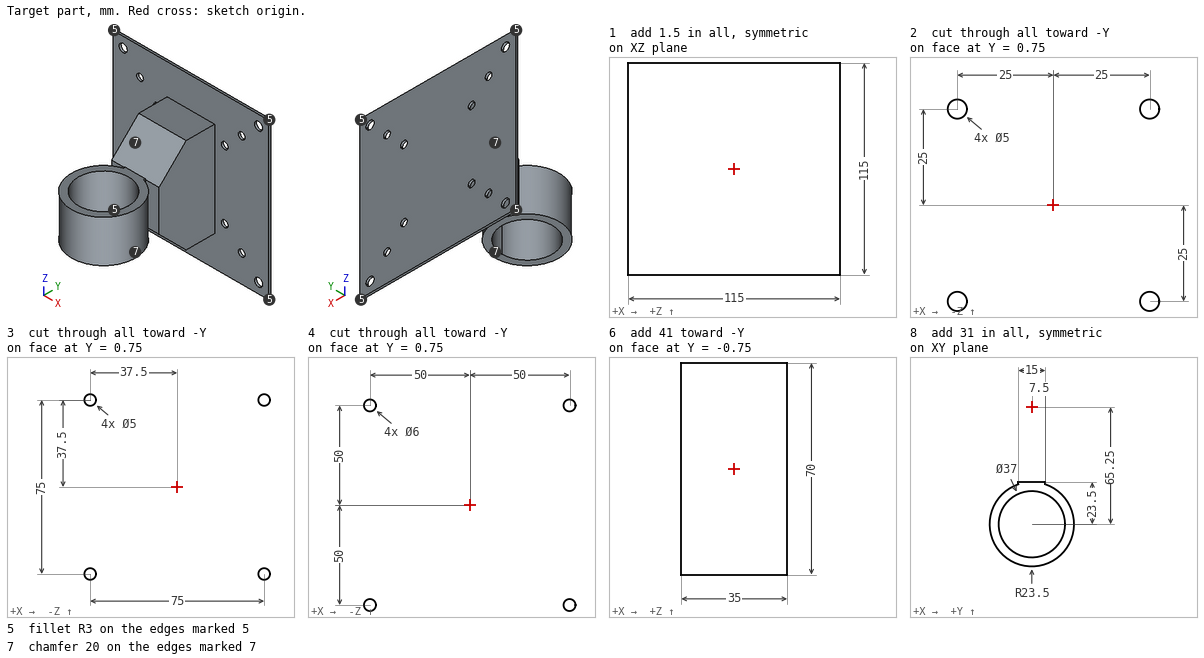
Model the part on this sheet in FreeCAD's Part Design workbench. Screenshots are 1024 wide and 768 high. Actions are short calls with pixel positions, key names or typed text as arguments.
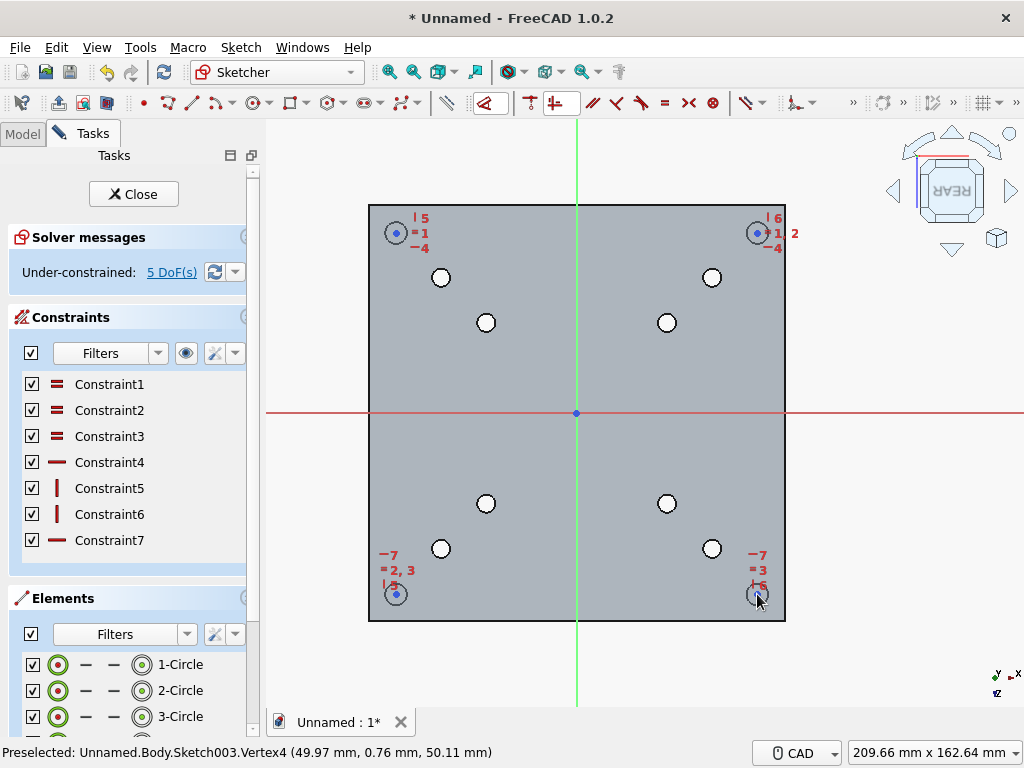
key(d)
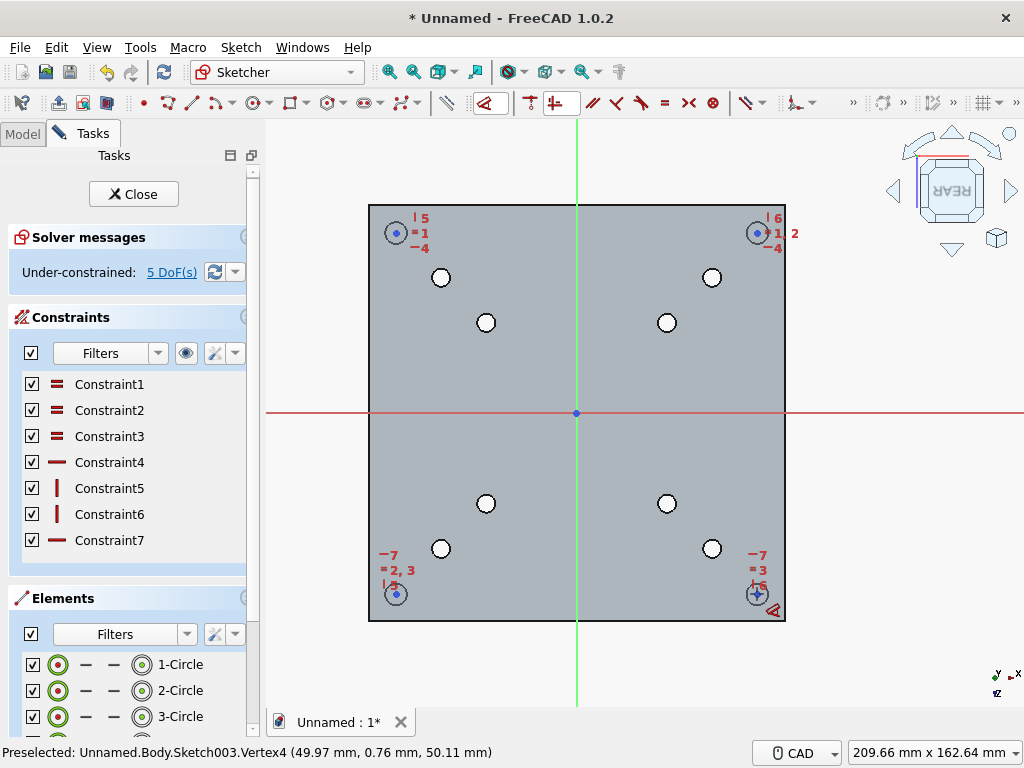
scroll(404, 225, up, 4)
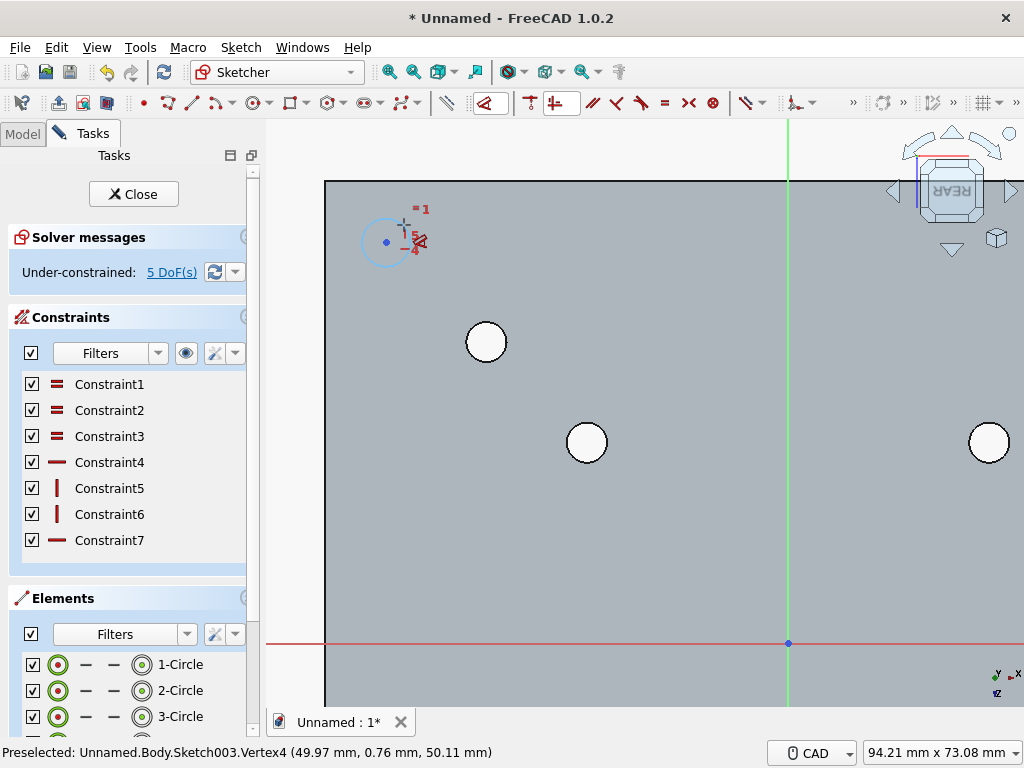
click(403, 226)
click(426, 203)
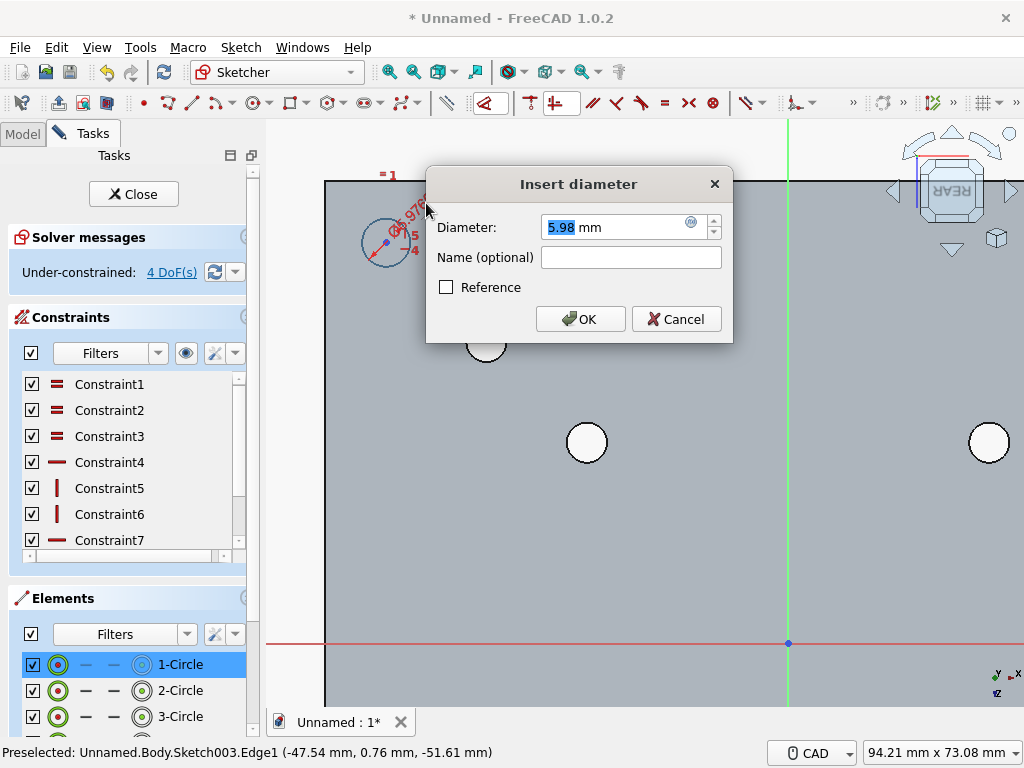
text(6)
key(Return)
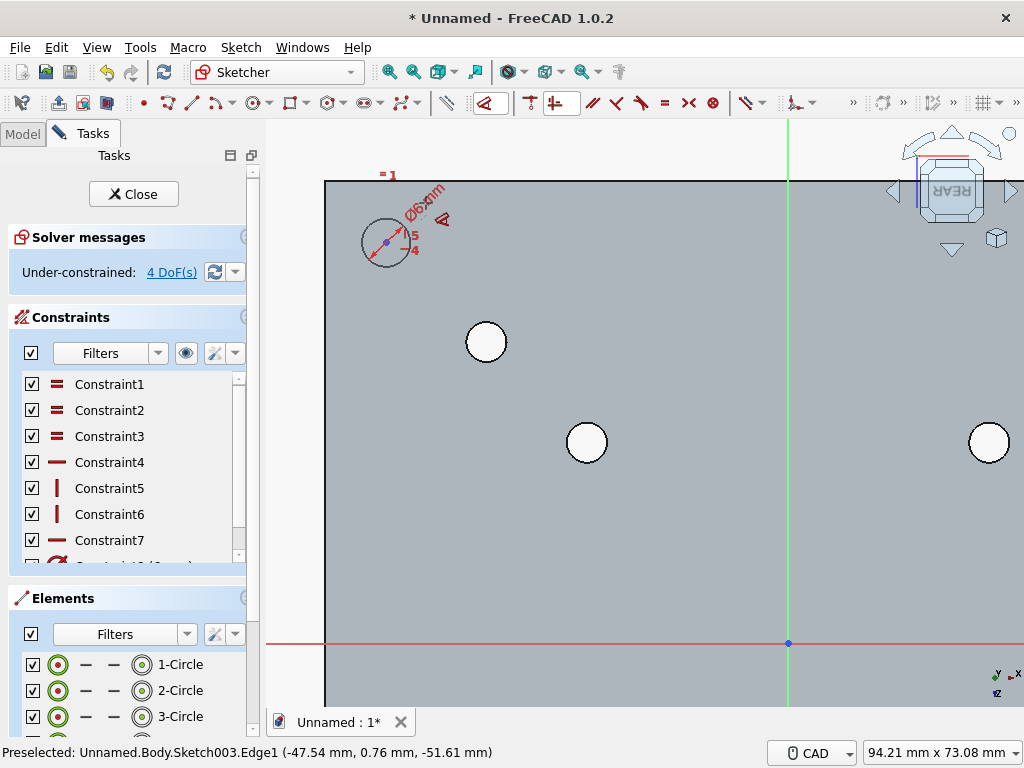
click(386, 243)
click(587, 209)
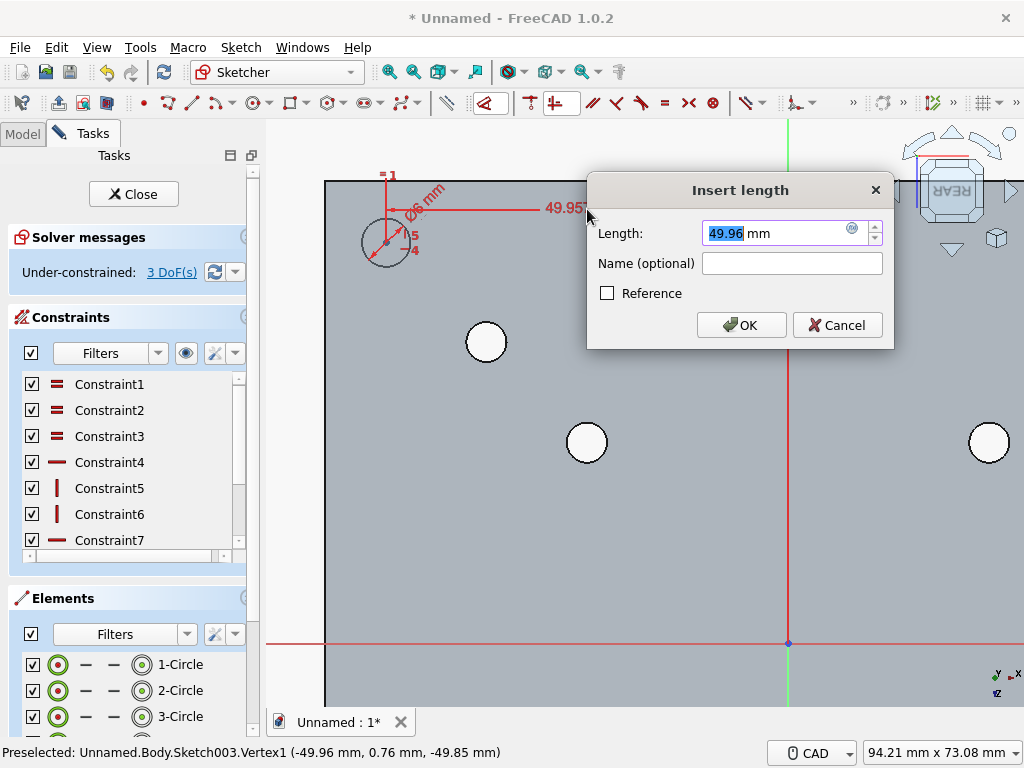
text(50)
key(Return)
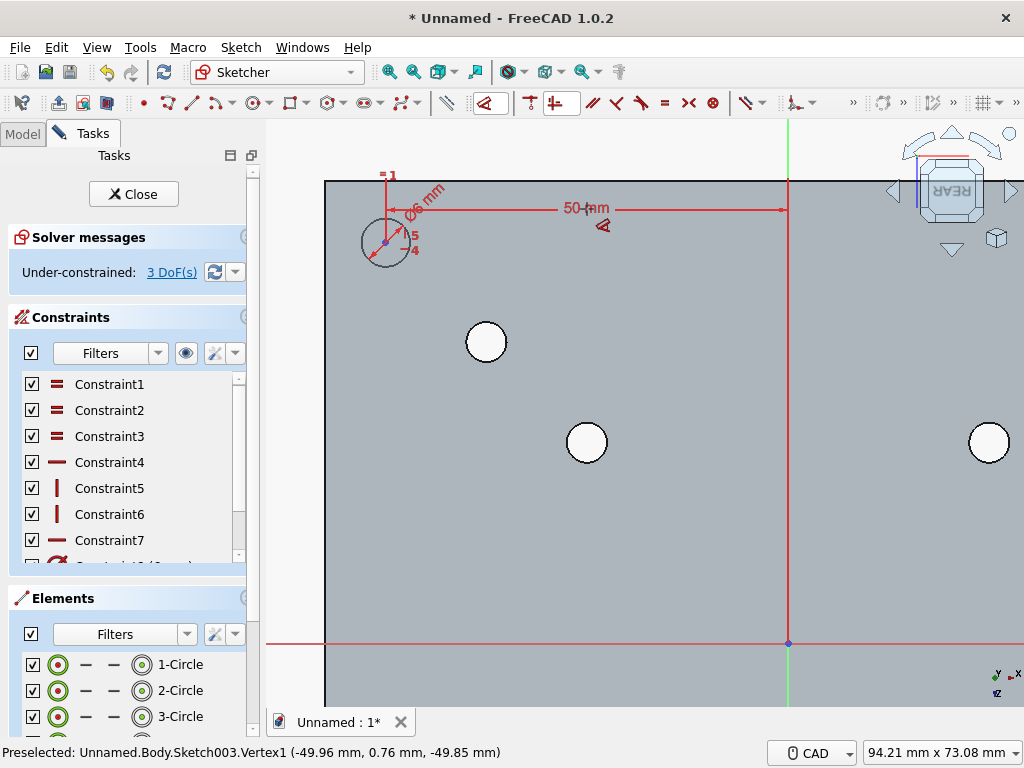
click(386, 243)
click(352, 443)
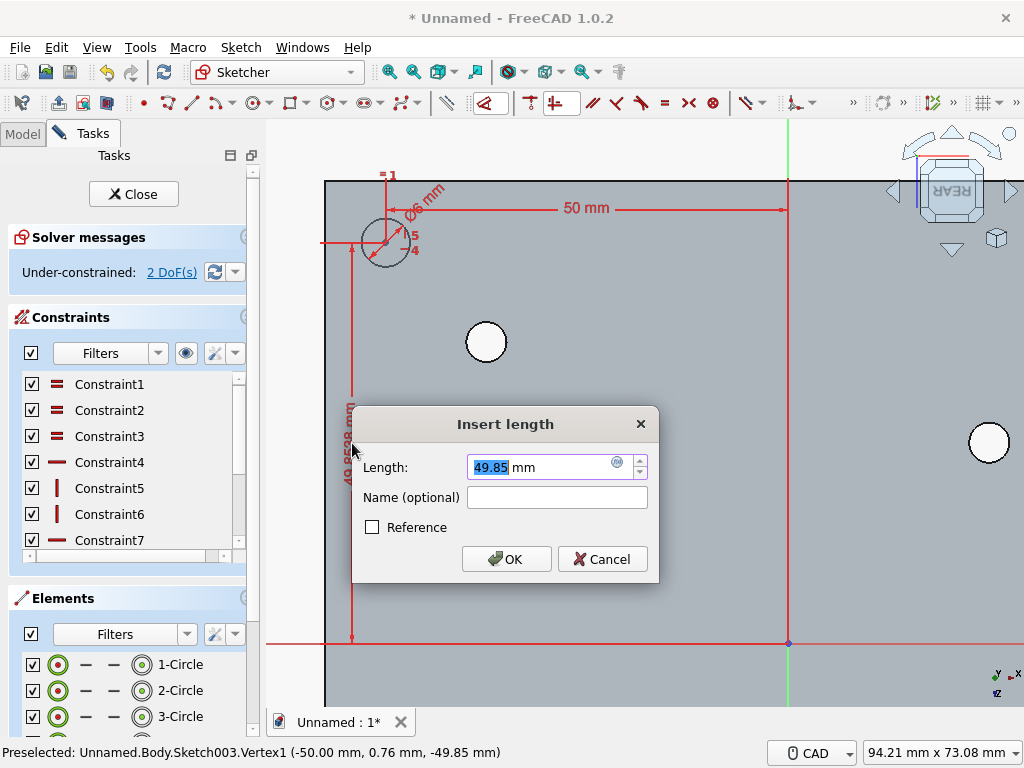
text(50)
key(Return)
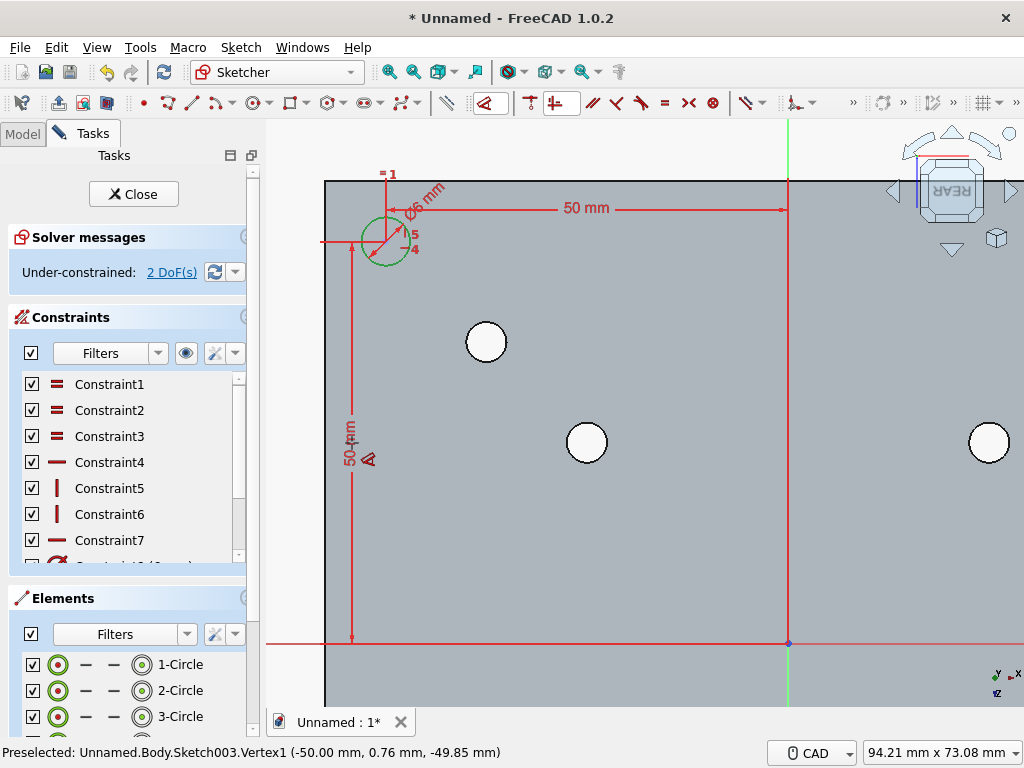
scroll(404, 225, down, 4)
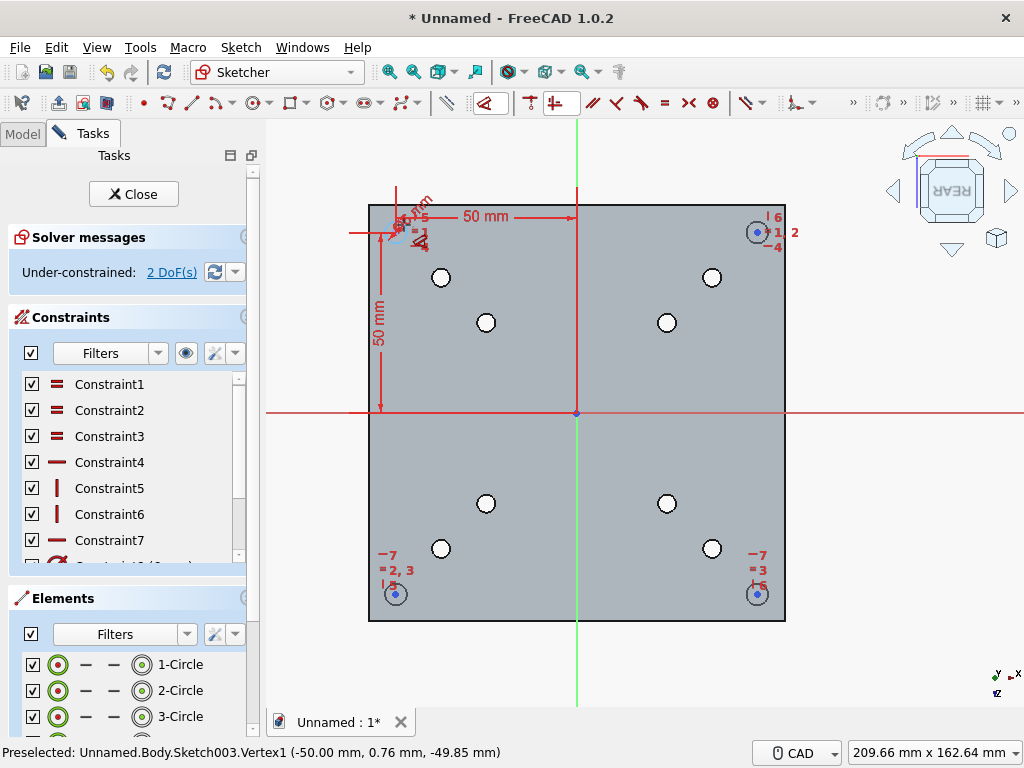
click(757, 233)
click(667, 199)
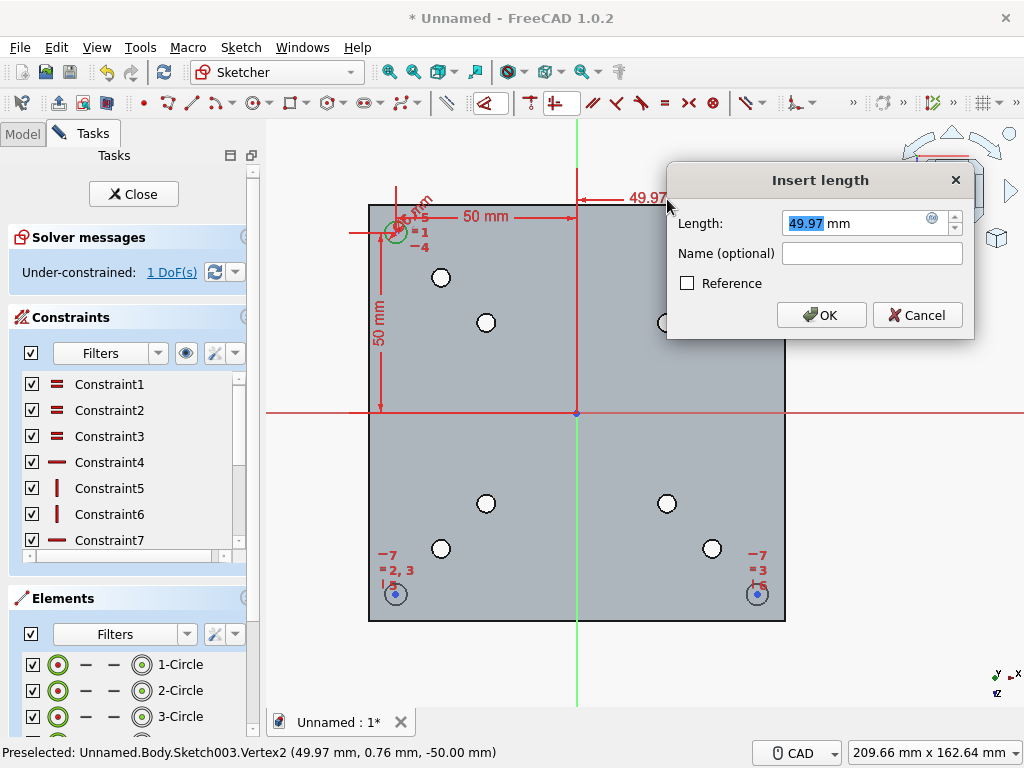
text(50)
key(Return)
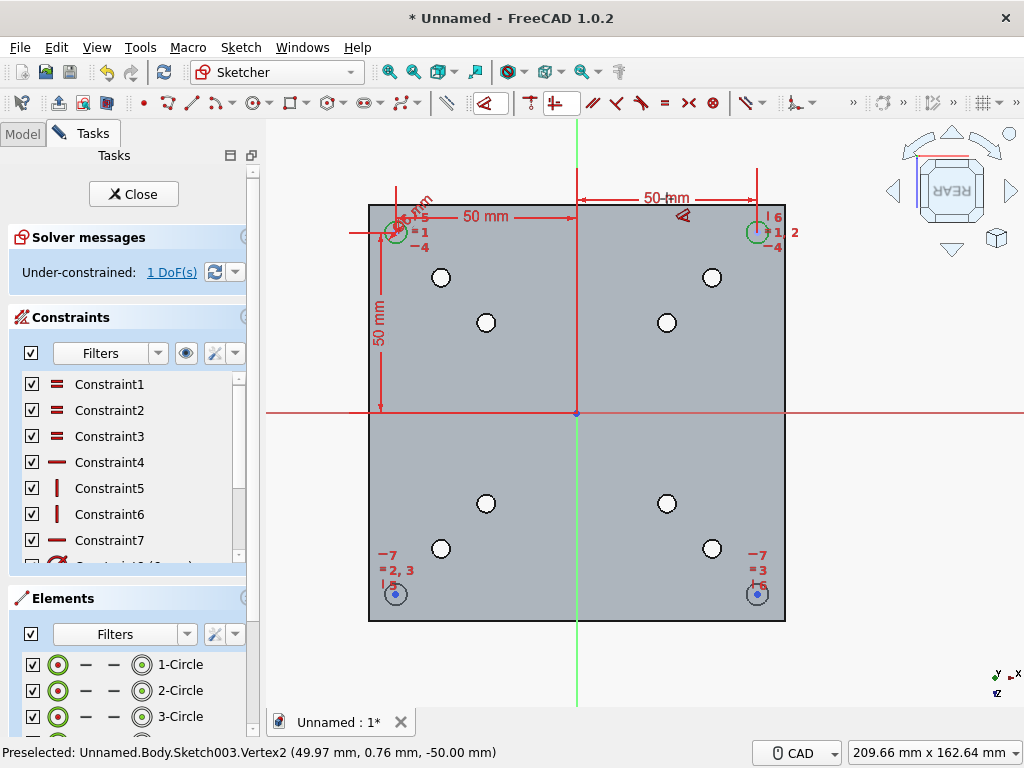
click(396, 594)
click(362, 504)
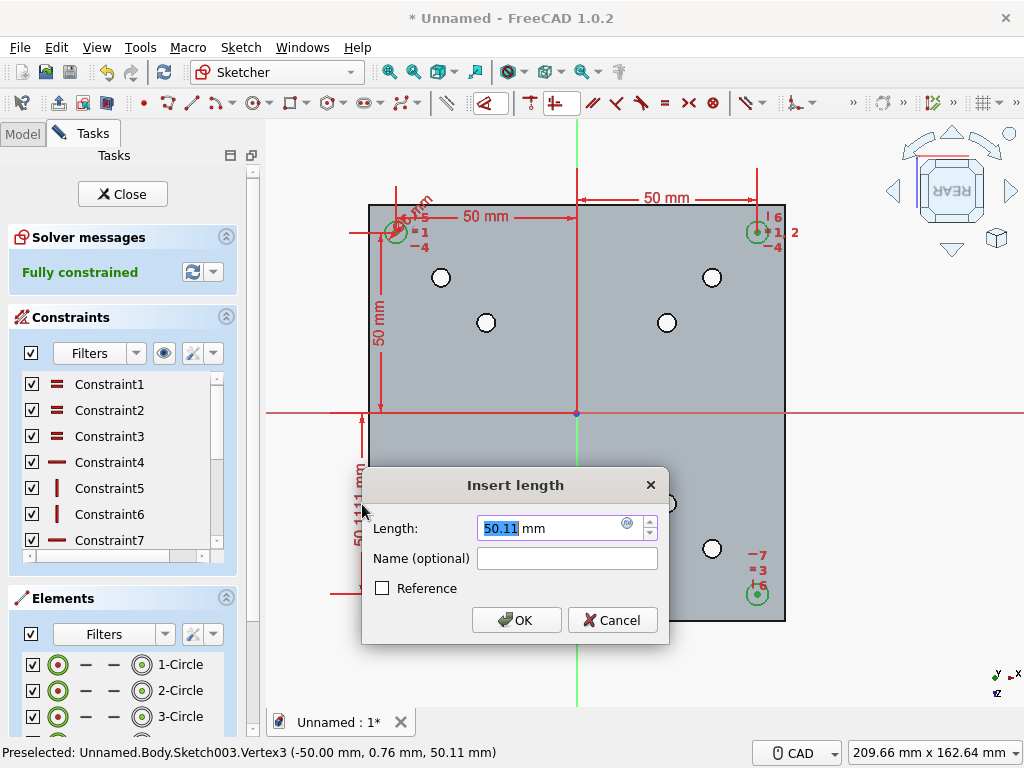
text(50)
key(Return)
key(Escape)